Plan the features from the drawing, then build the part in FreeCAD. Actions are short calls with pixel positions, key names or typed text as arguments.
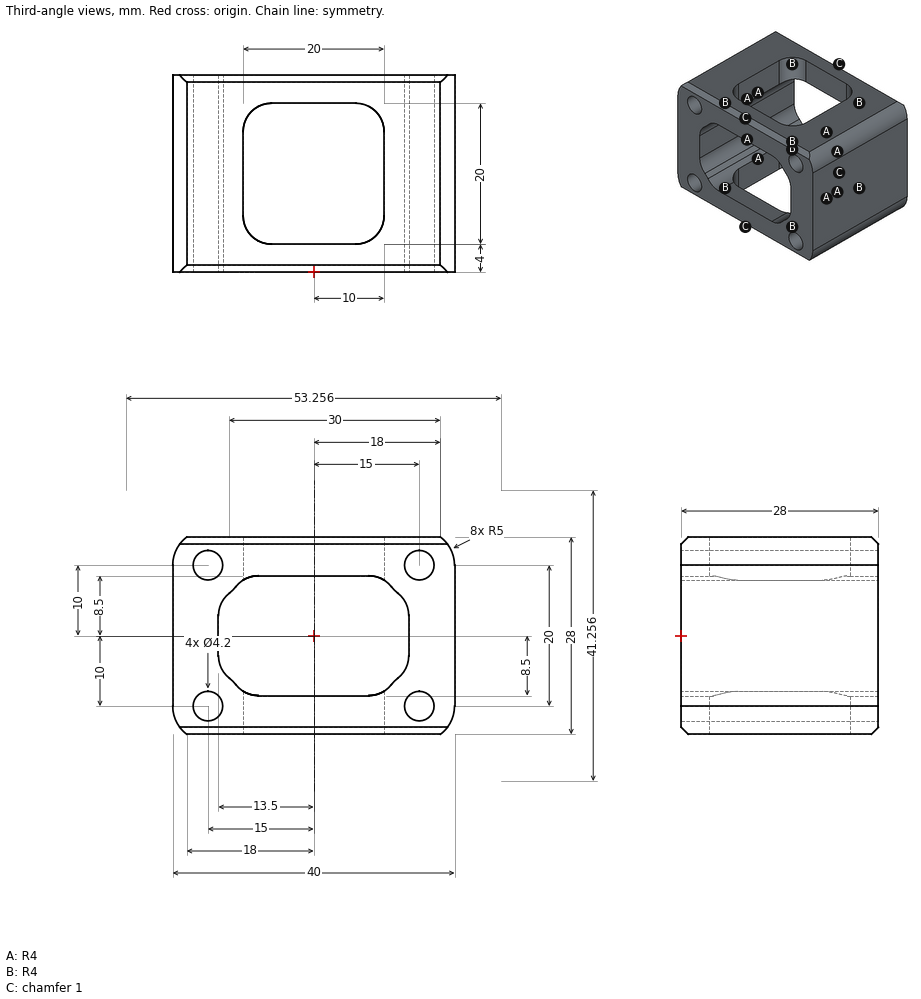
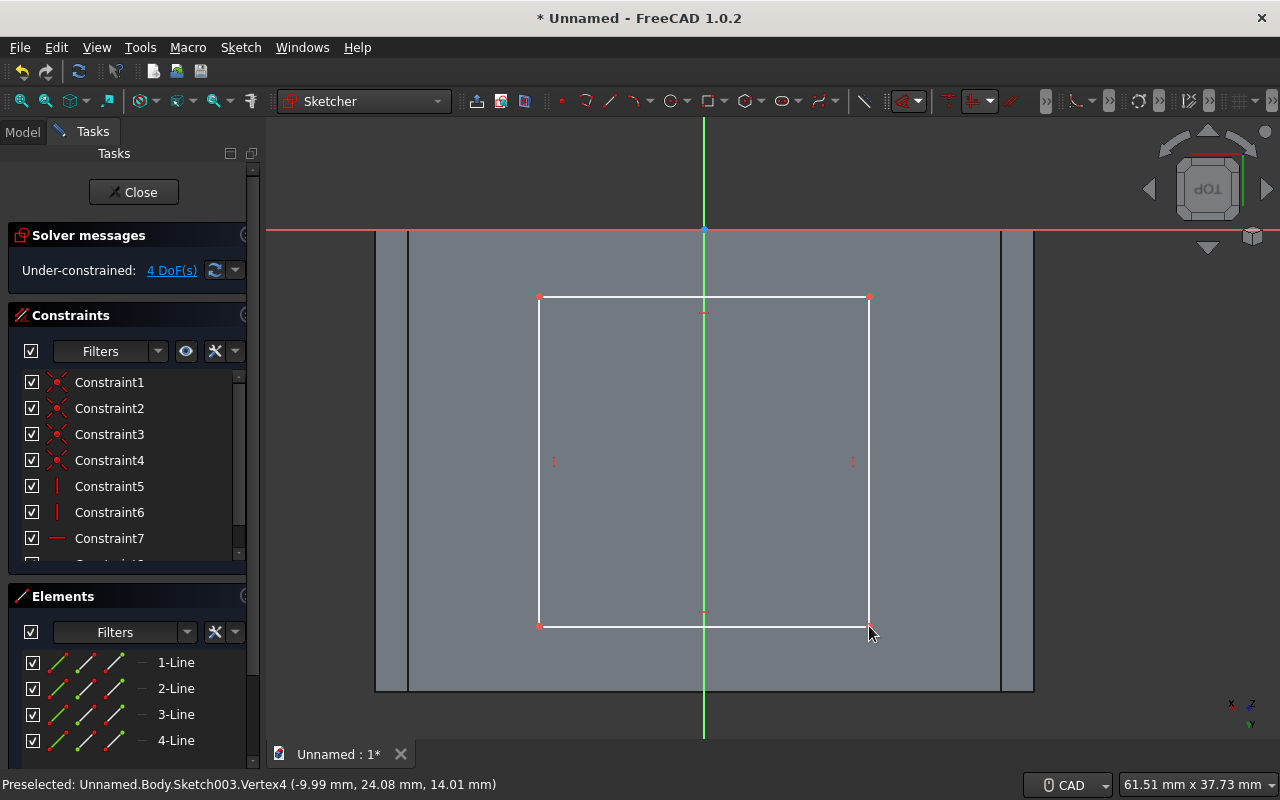
click(539, 396)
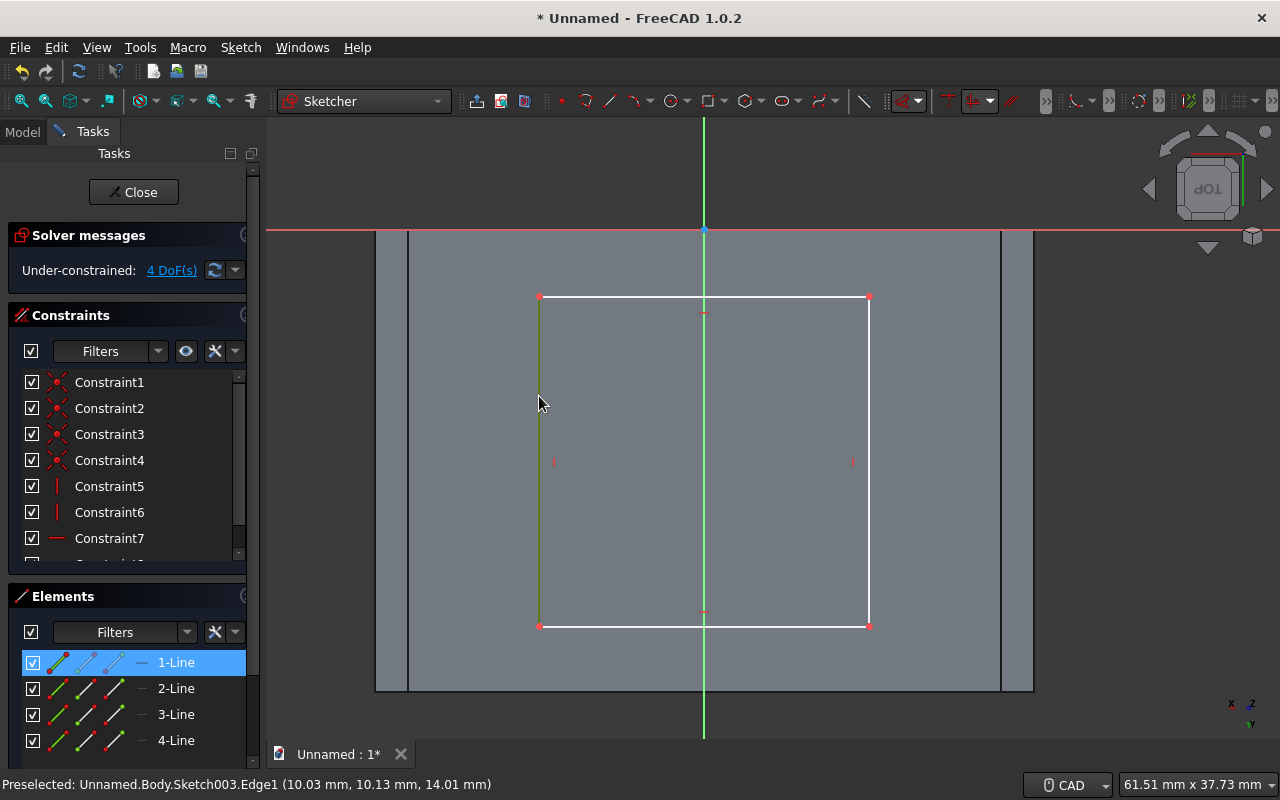
key(i)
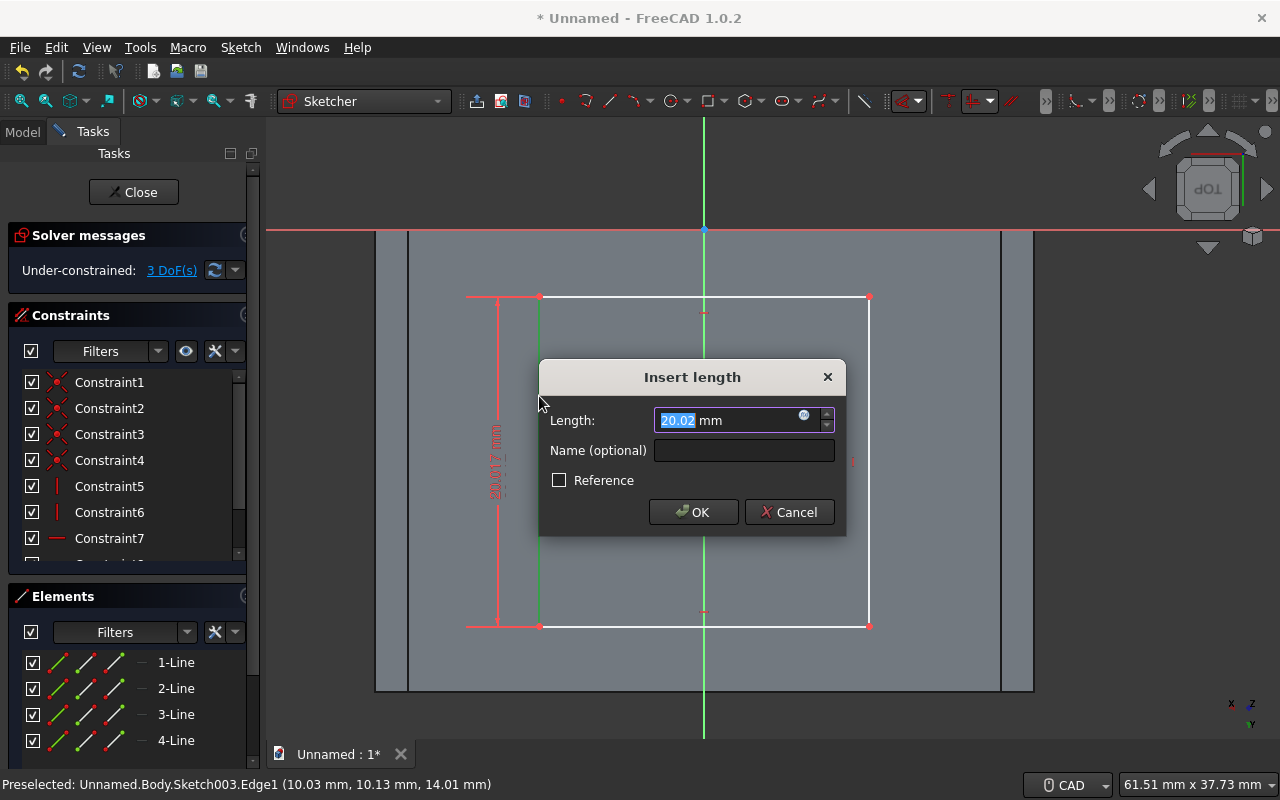
text(20)
key(Return)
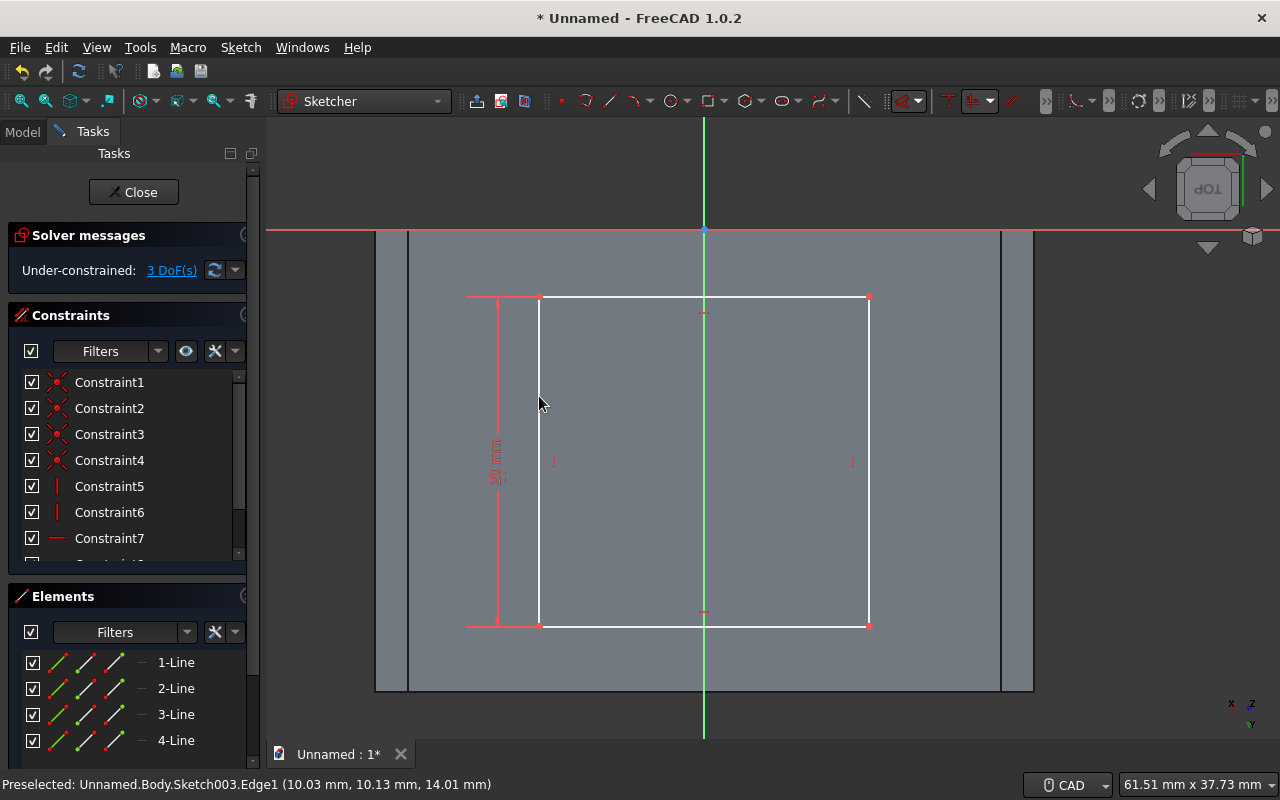
click(638, 627)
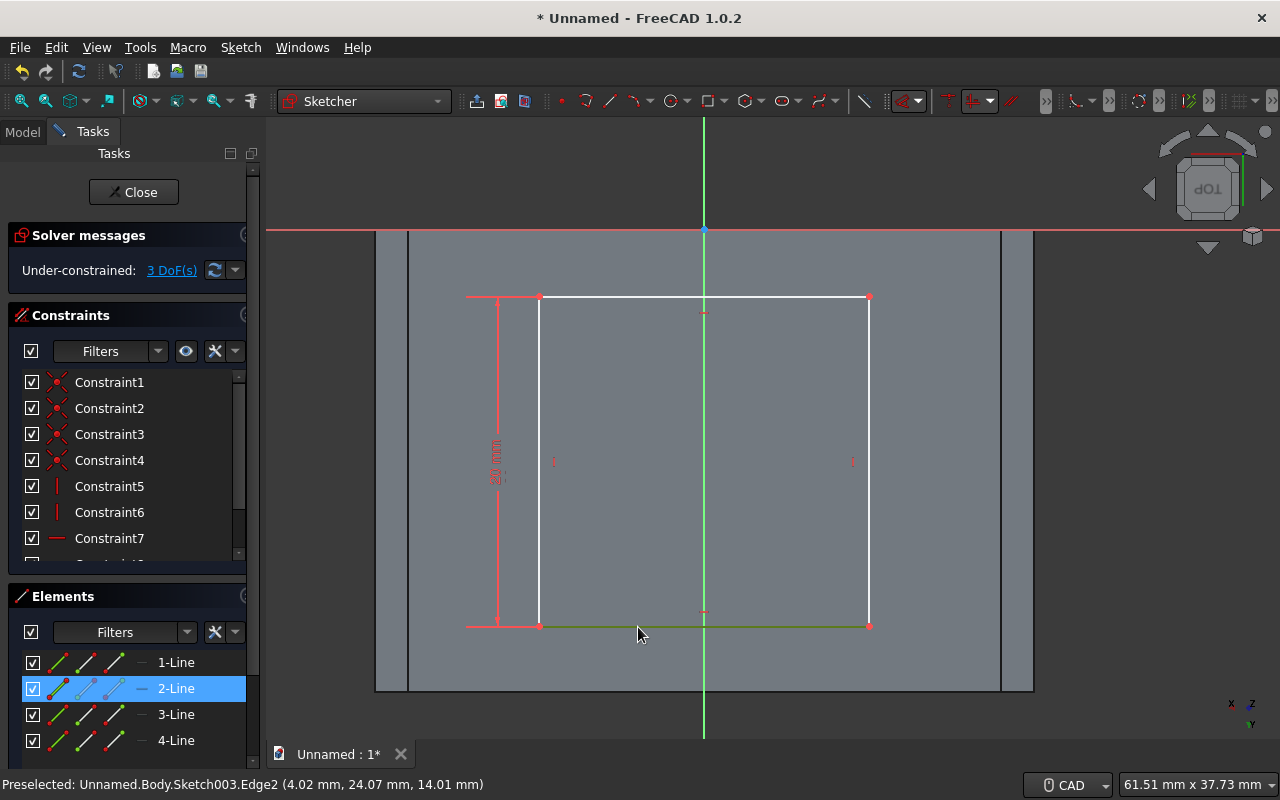
key(l)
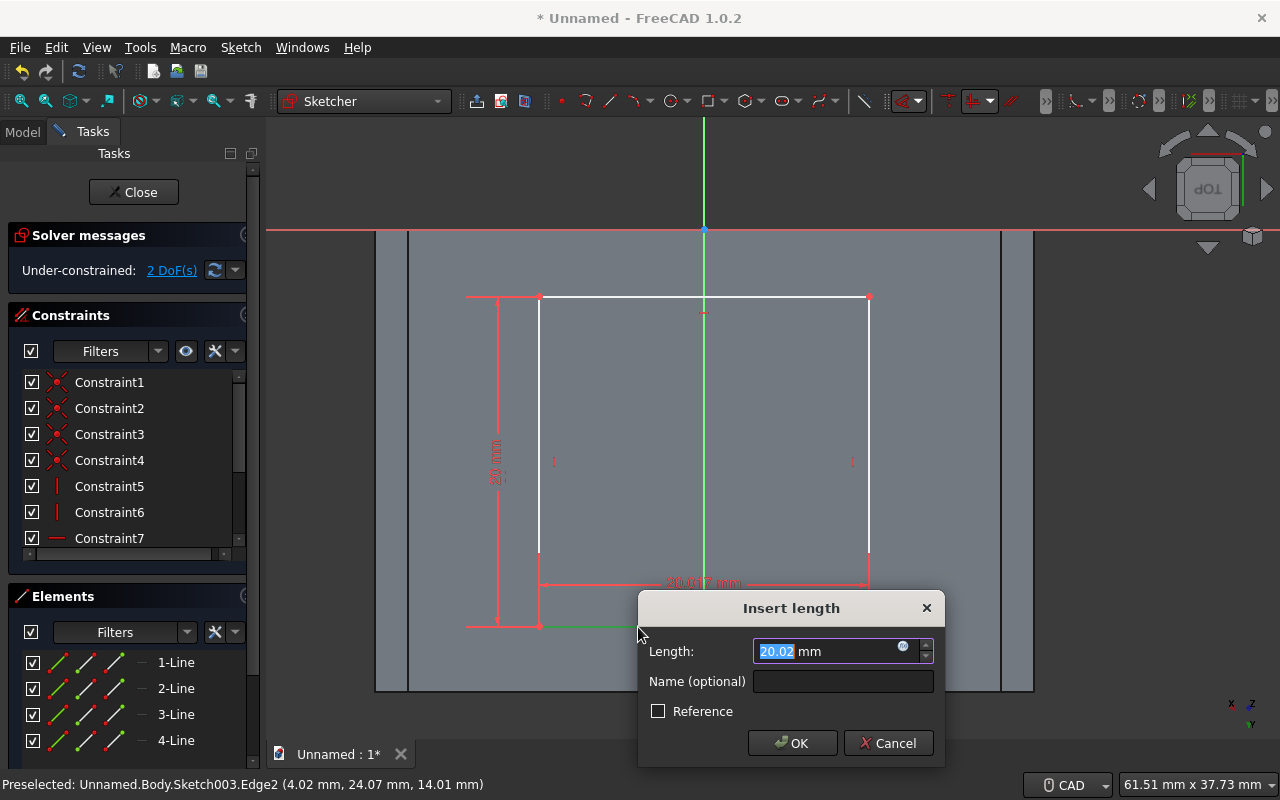
text(20)
key(Return)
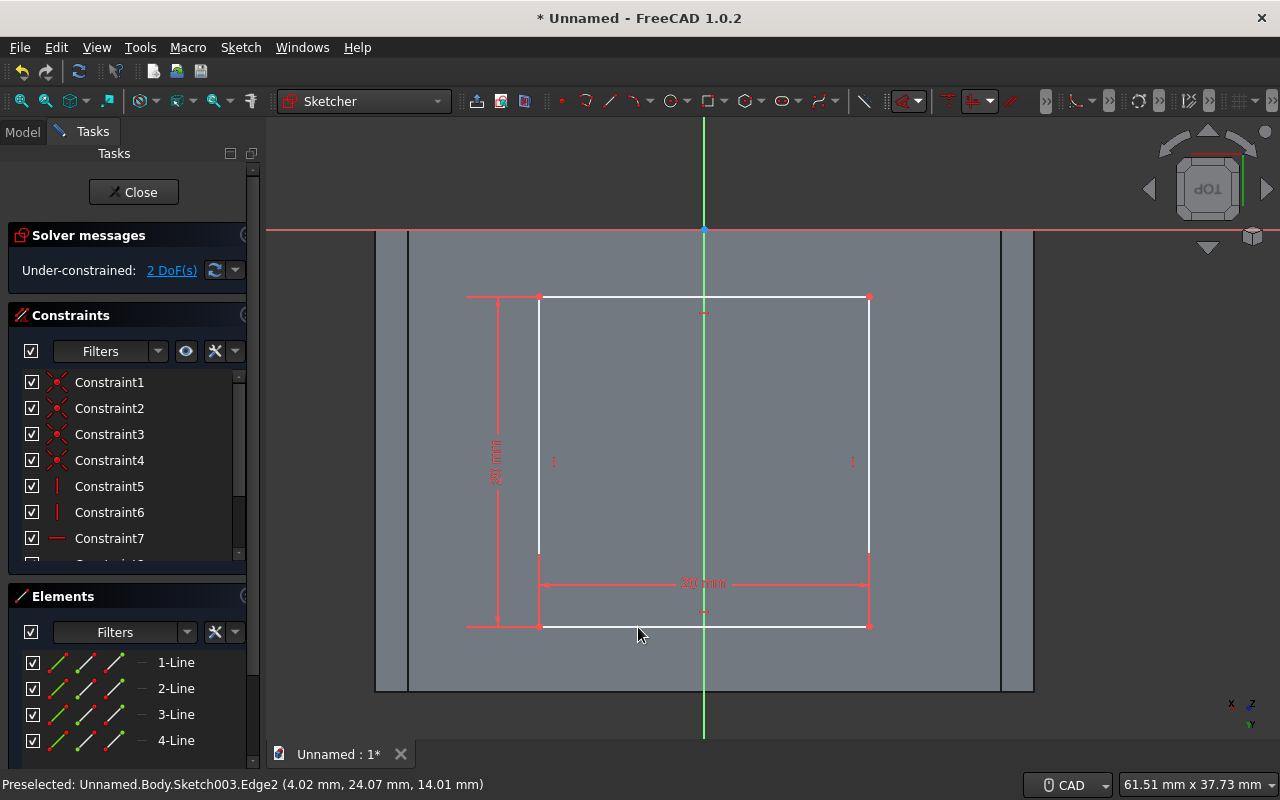
click(539, 297)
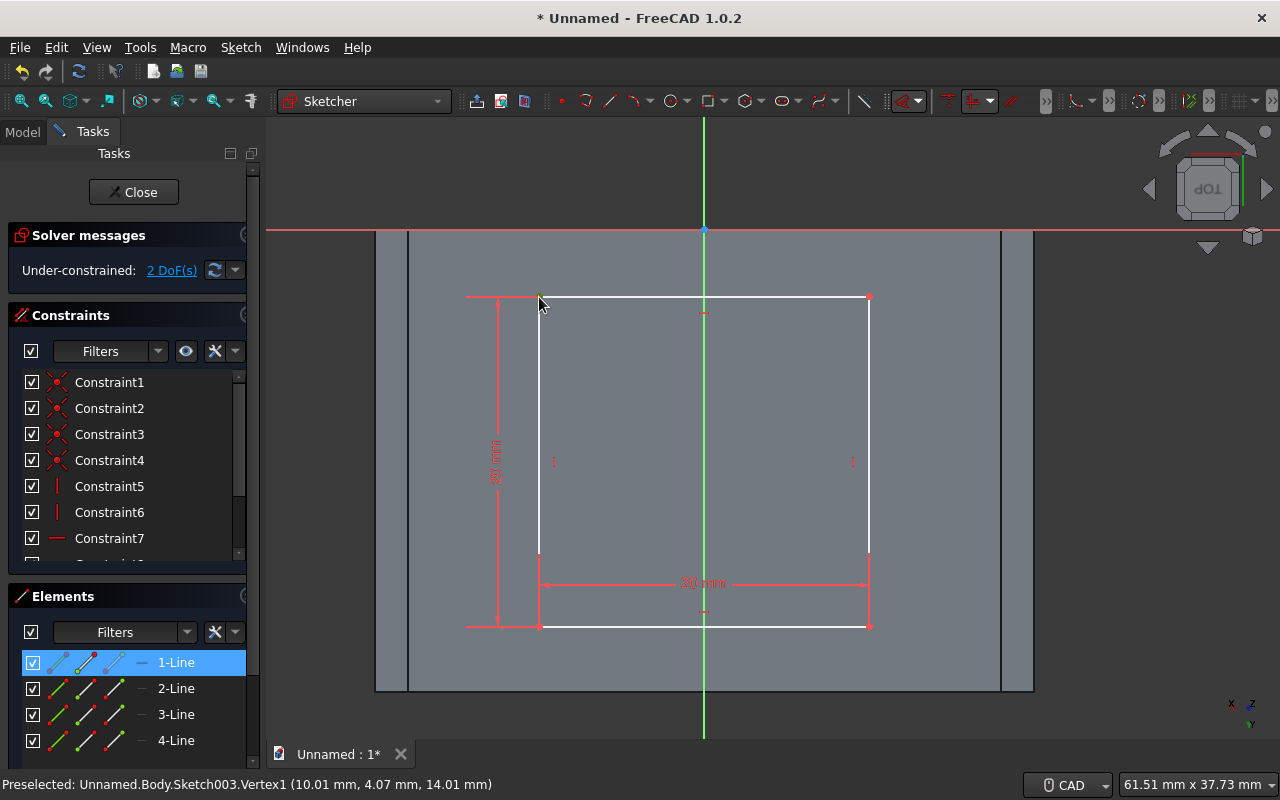
key(i)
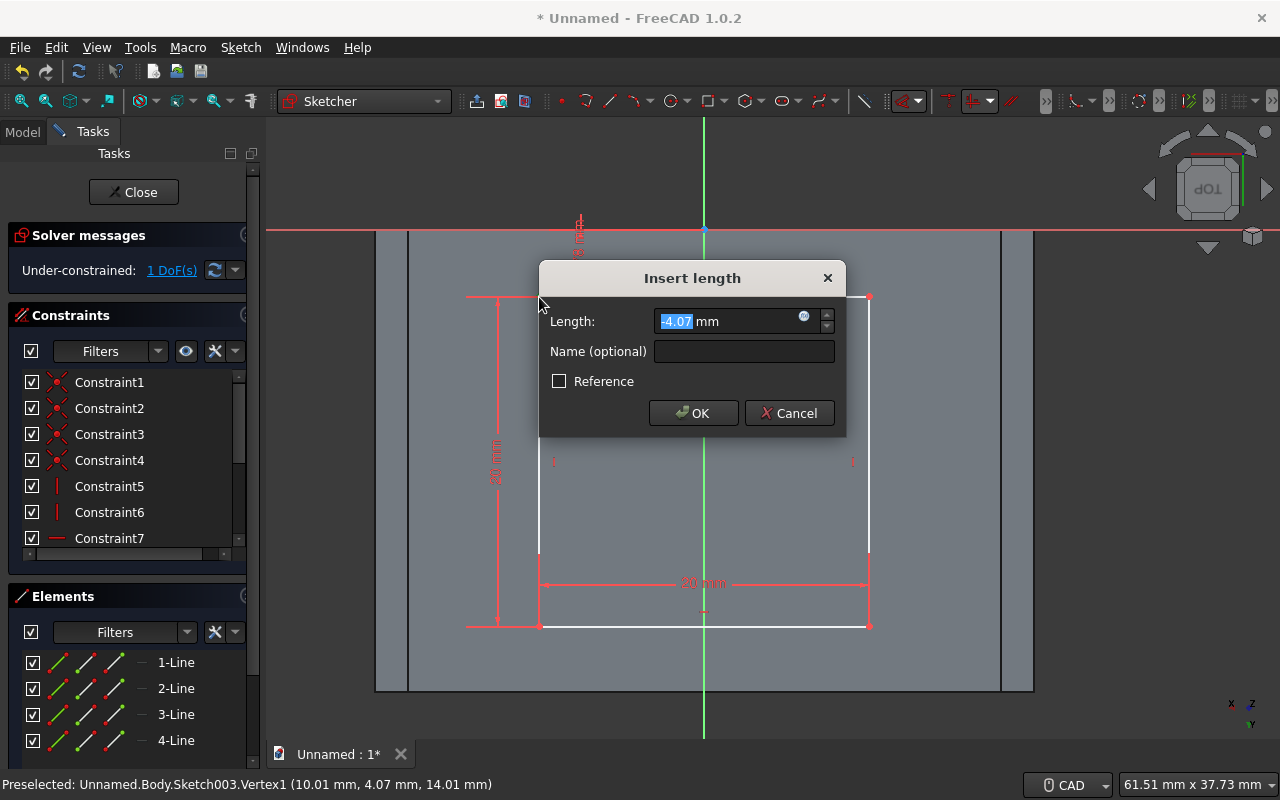
text(-4)
key(Return)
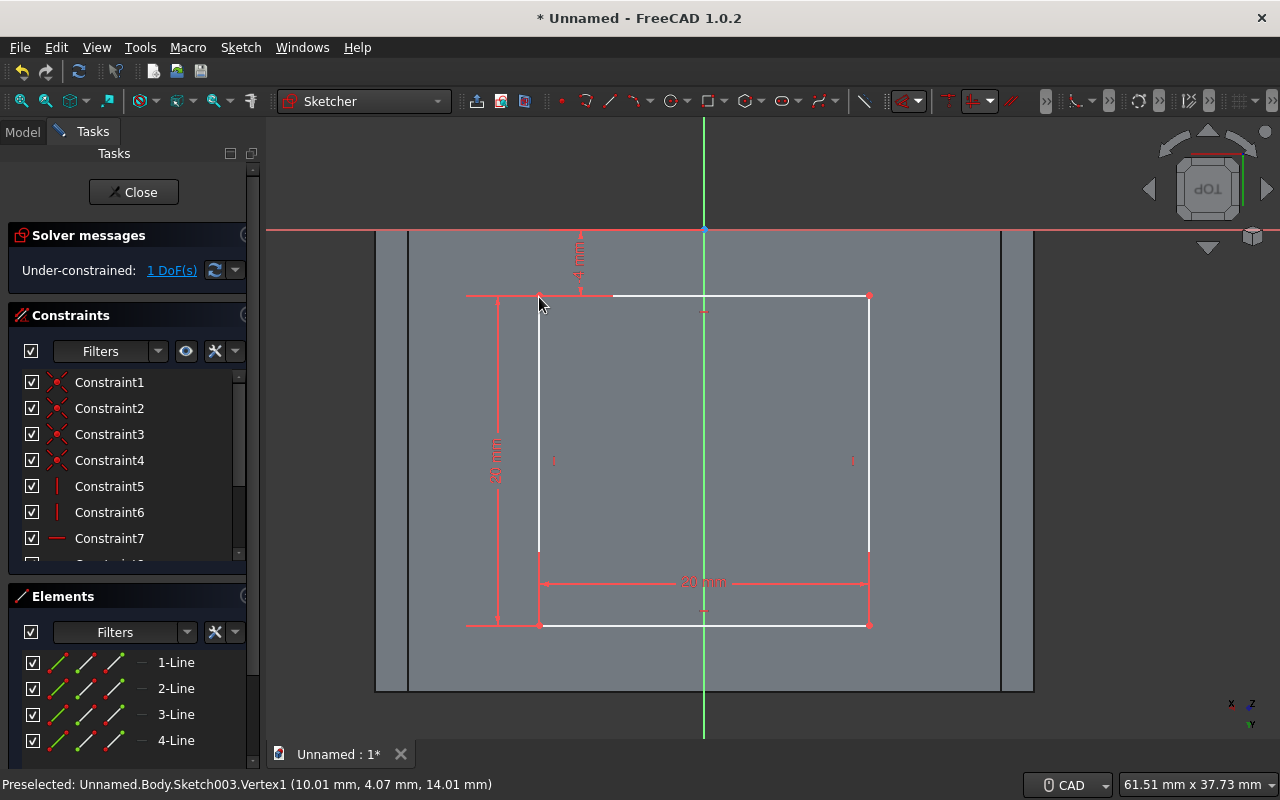
click(539, 296)